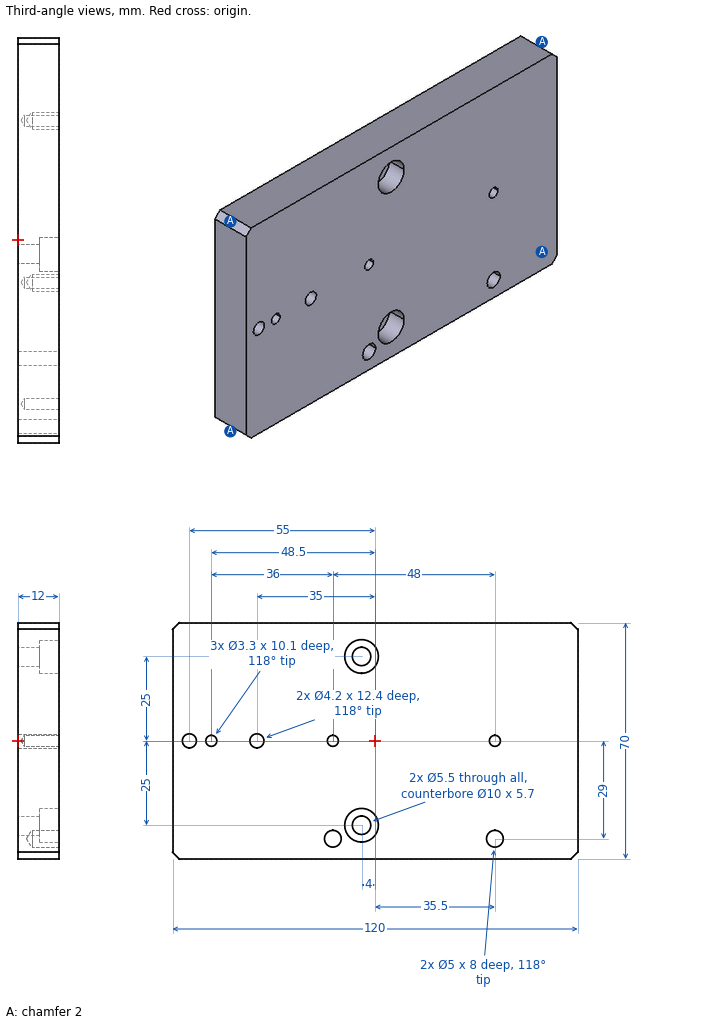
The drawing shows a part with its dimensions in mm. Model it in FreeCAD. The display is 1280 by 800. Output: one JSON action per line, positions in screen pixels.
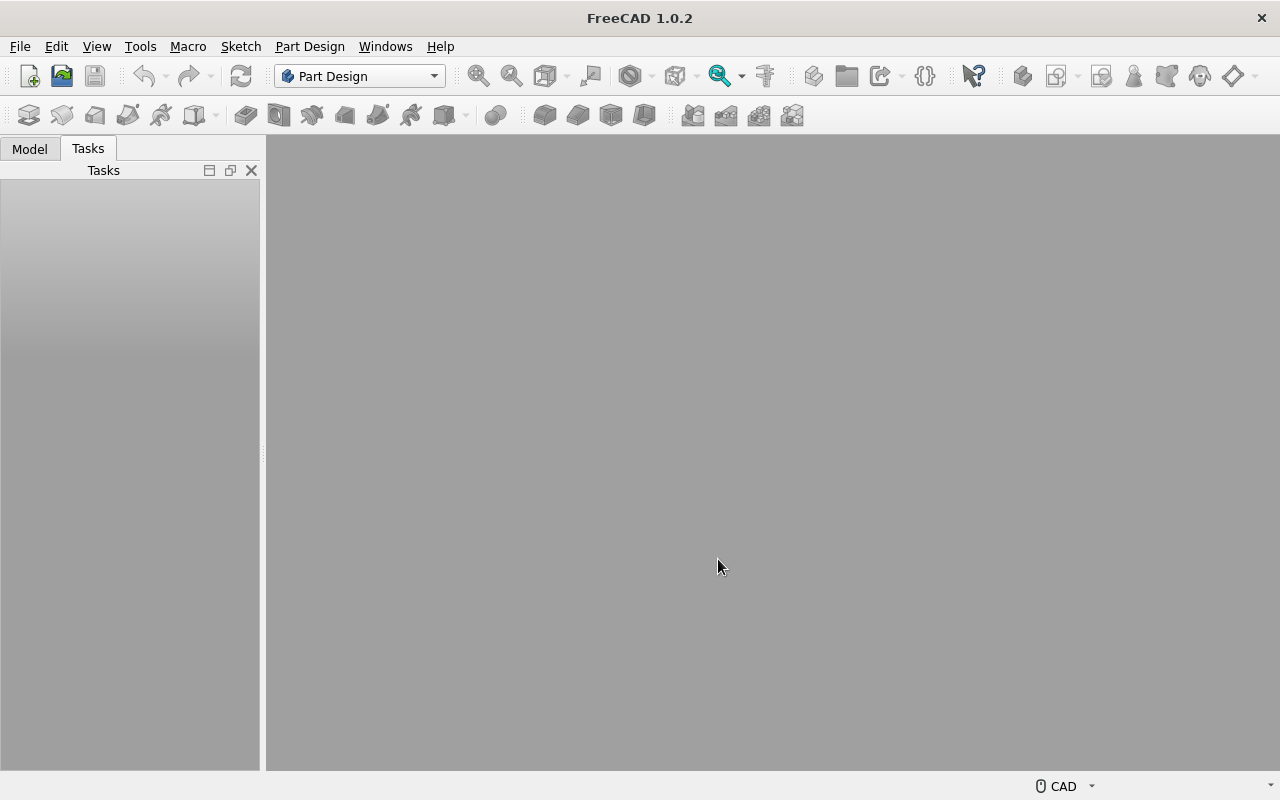
{"action": "left_click", "coordinate": [29, 76]}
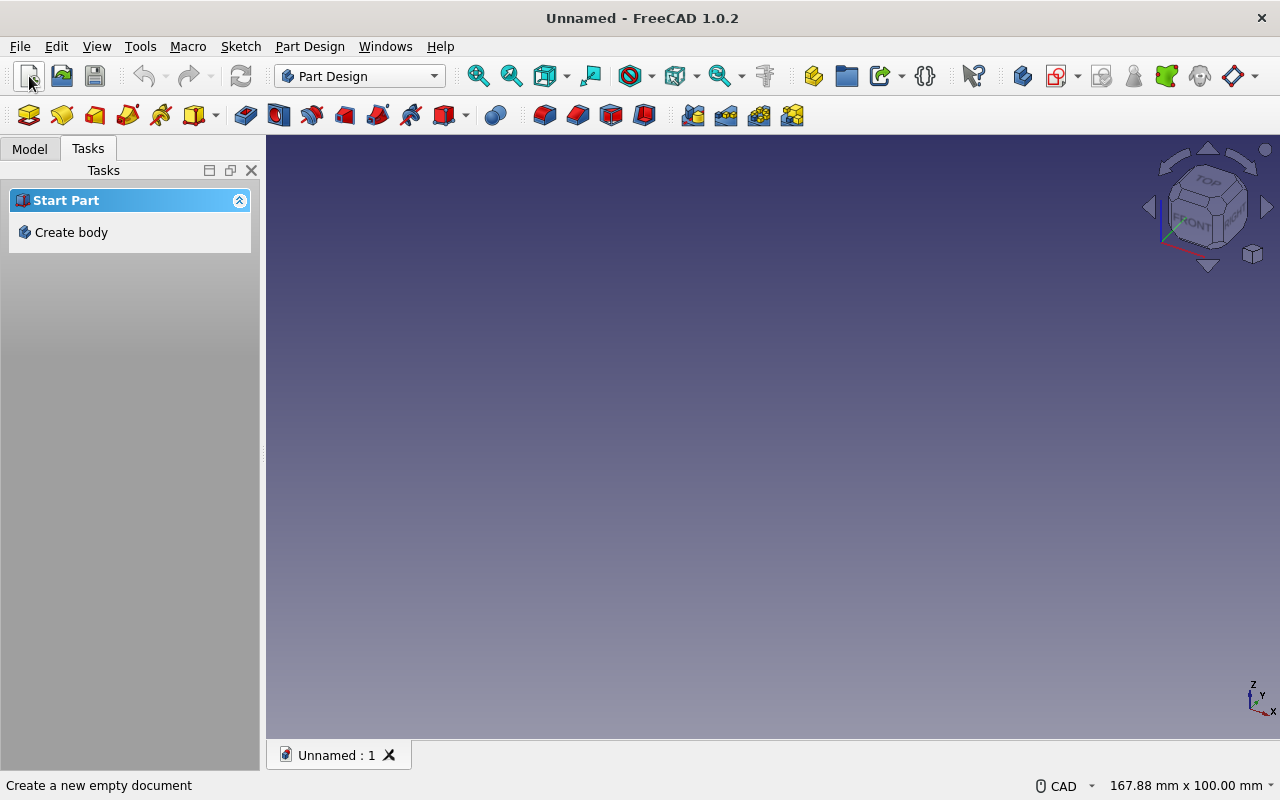
{"action": "left_click", "coordinate": [1056, 76]}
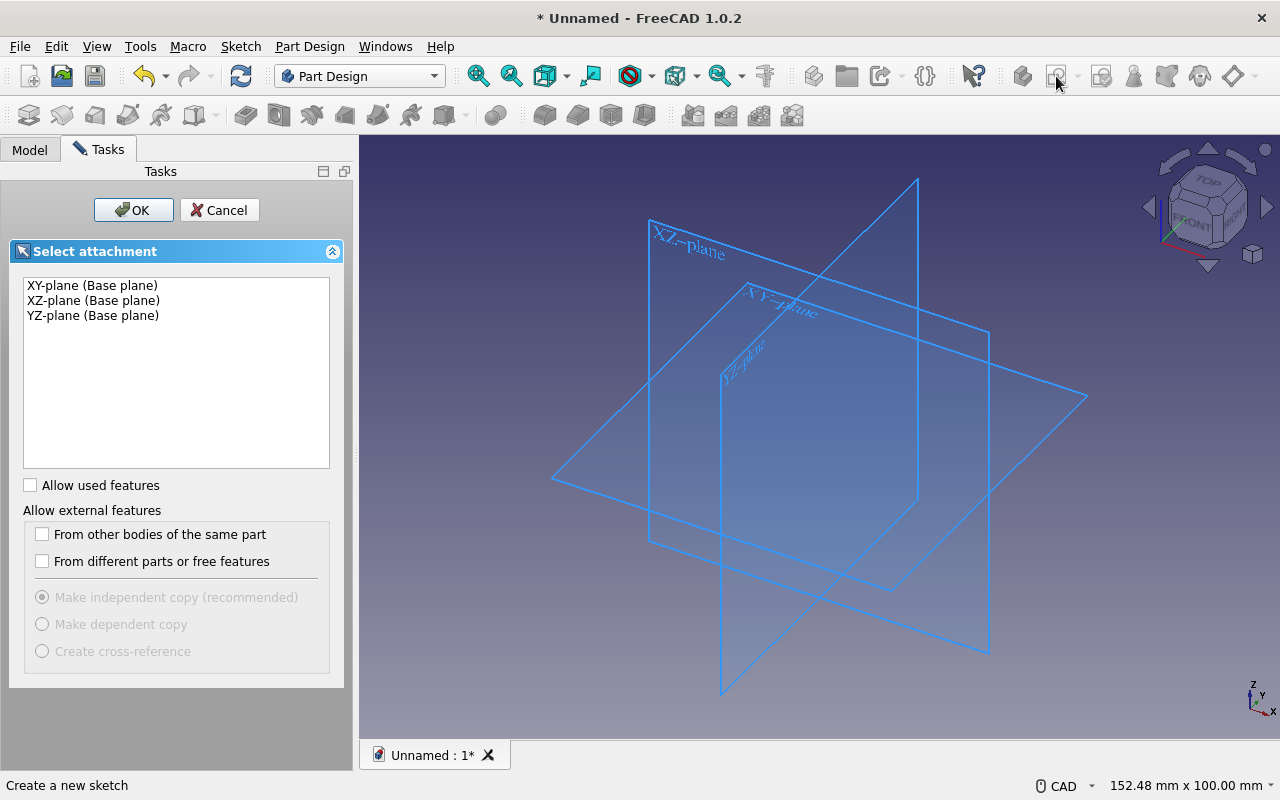
{"action": "left_click", "coordinate": [84, 316]}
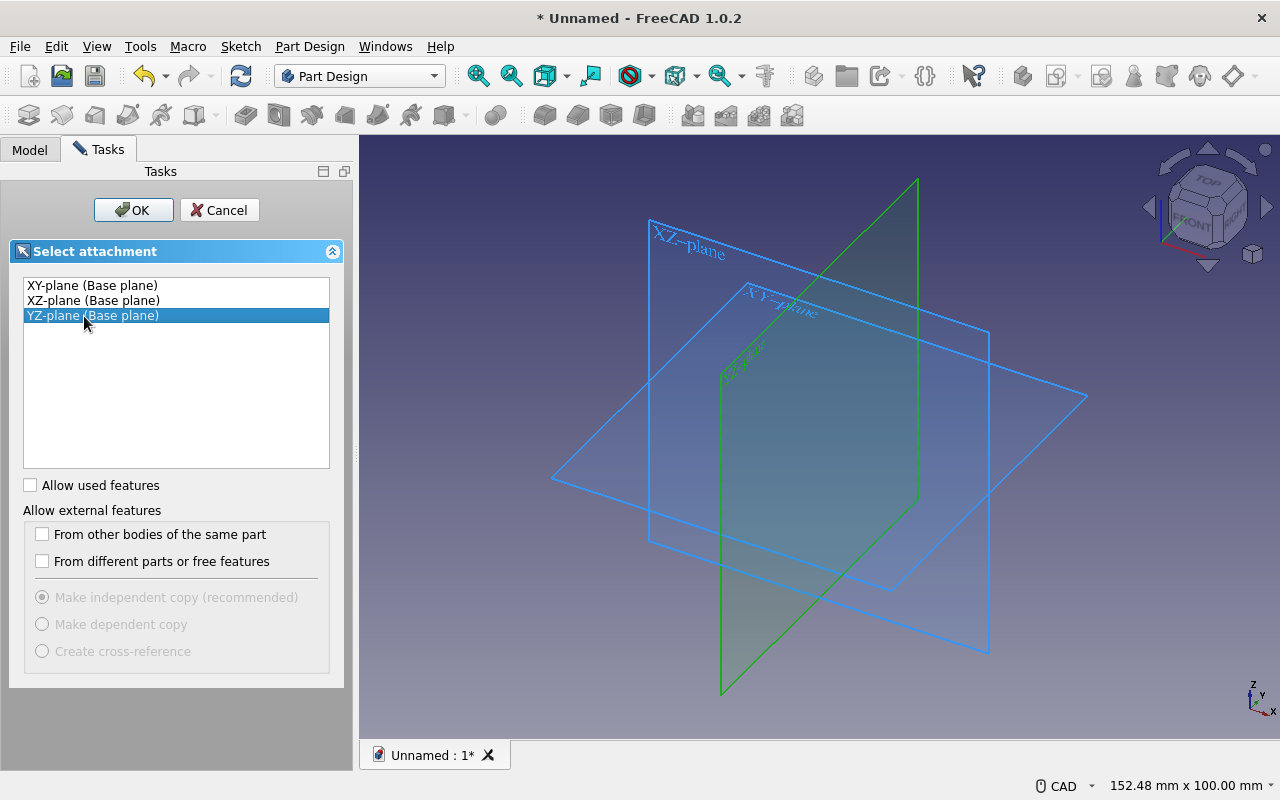
{"action": "left_click", "coordinate": [134, 210]}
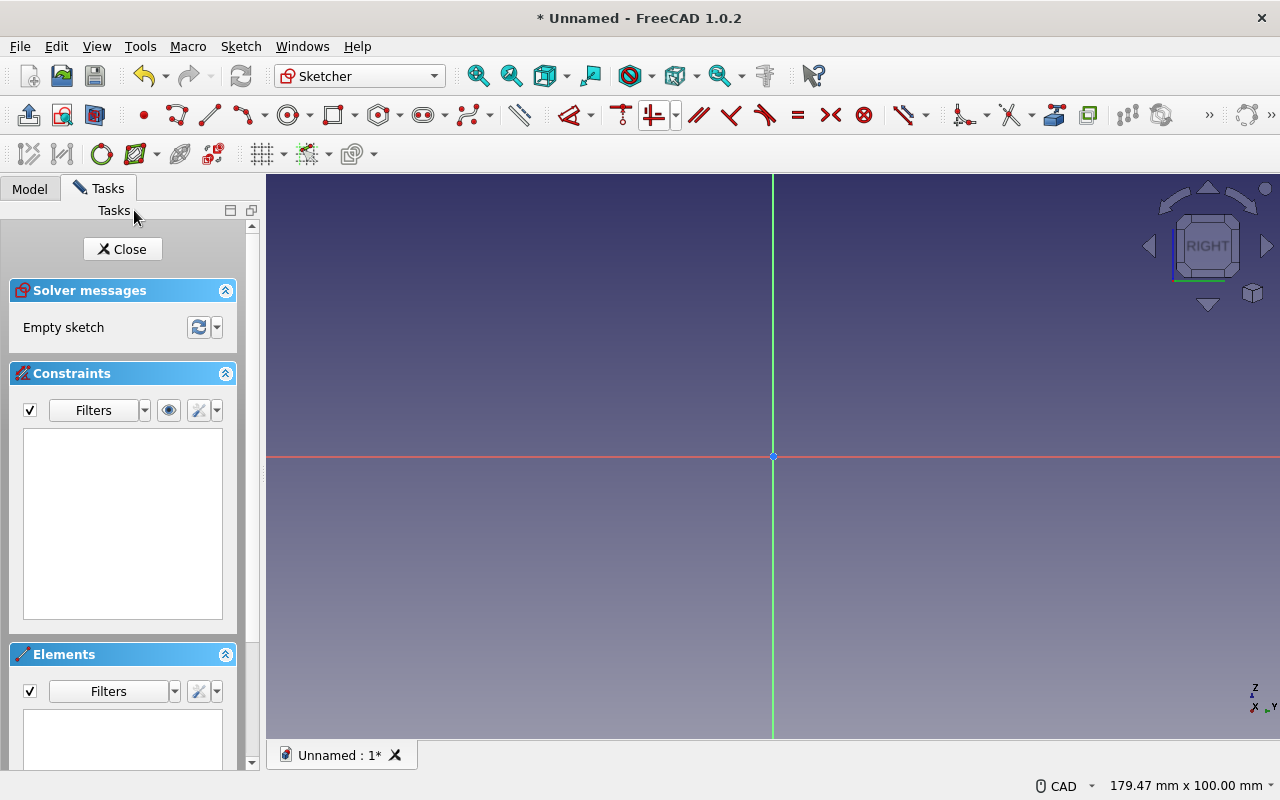
{"action": "scroll", "coordinate": [395, 456], "scroll_direction": "down", "scroll_amount": 1}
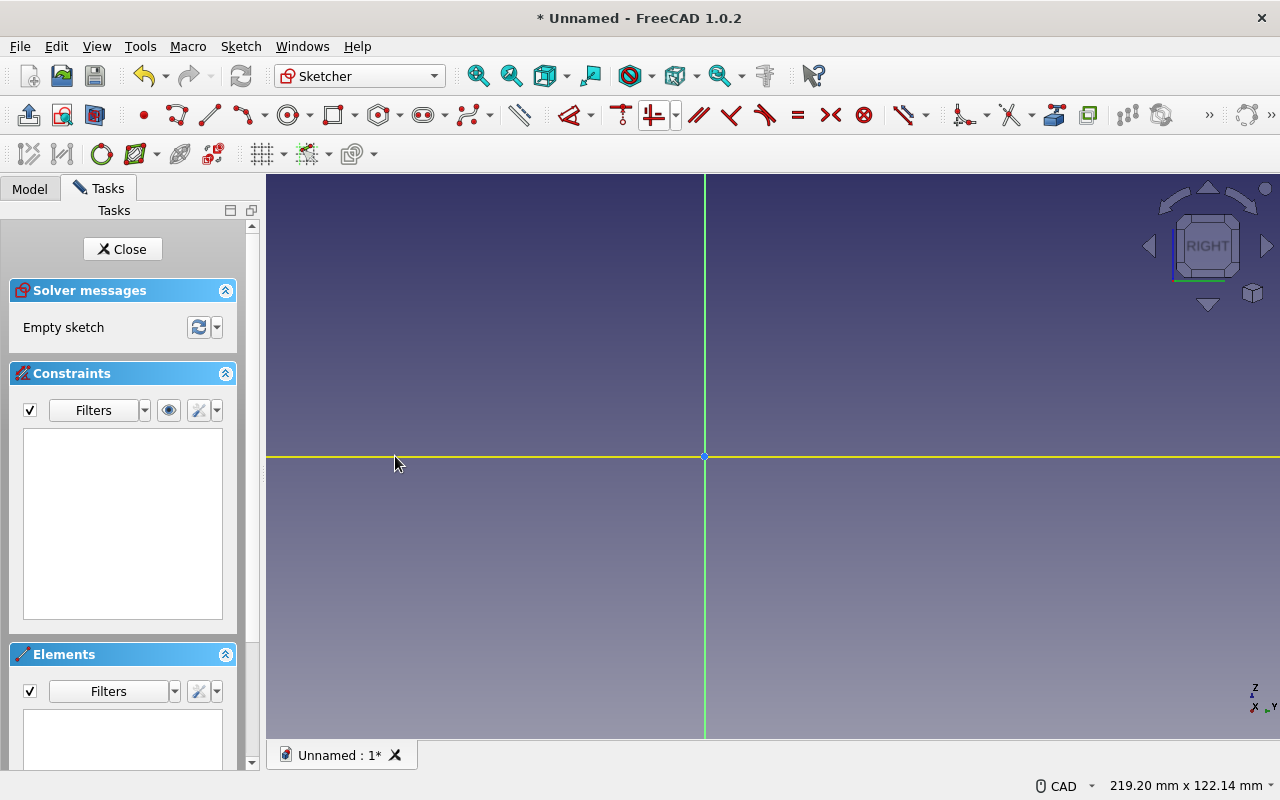
{"action": "key", "text": "g v"}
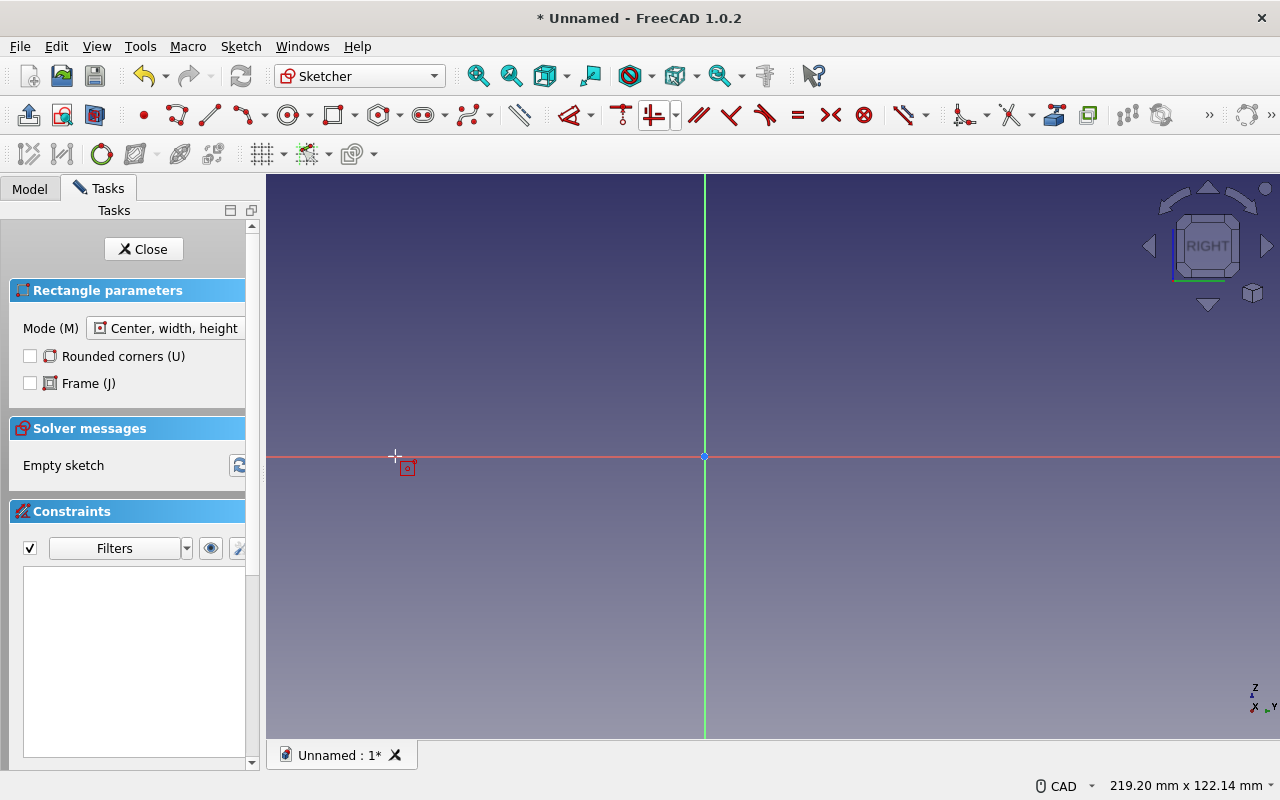
{"action": "left_click", "coordinate": [705, 456]}
{"action": "left_click", "coordinate": [982, 295]}
{"action": "key", "text": "Escape"}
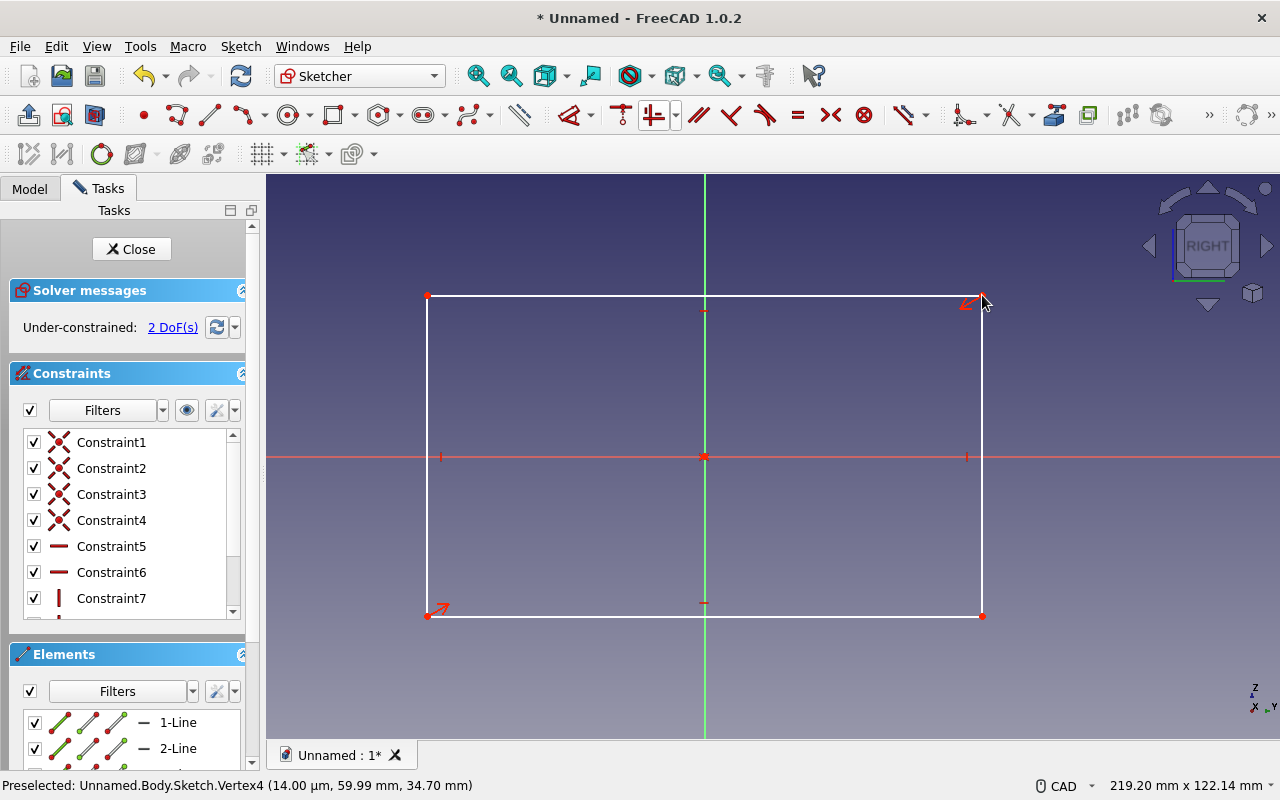
{"action": "left_click", "coordinate": [568, 116]}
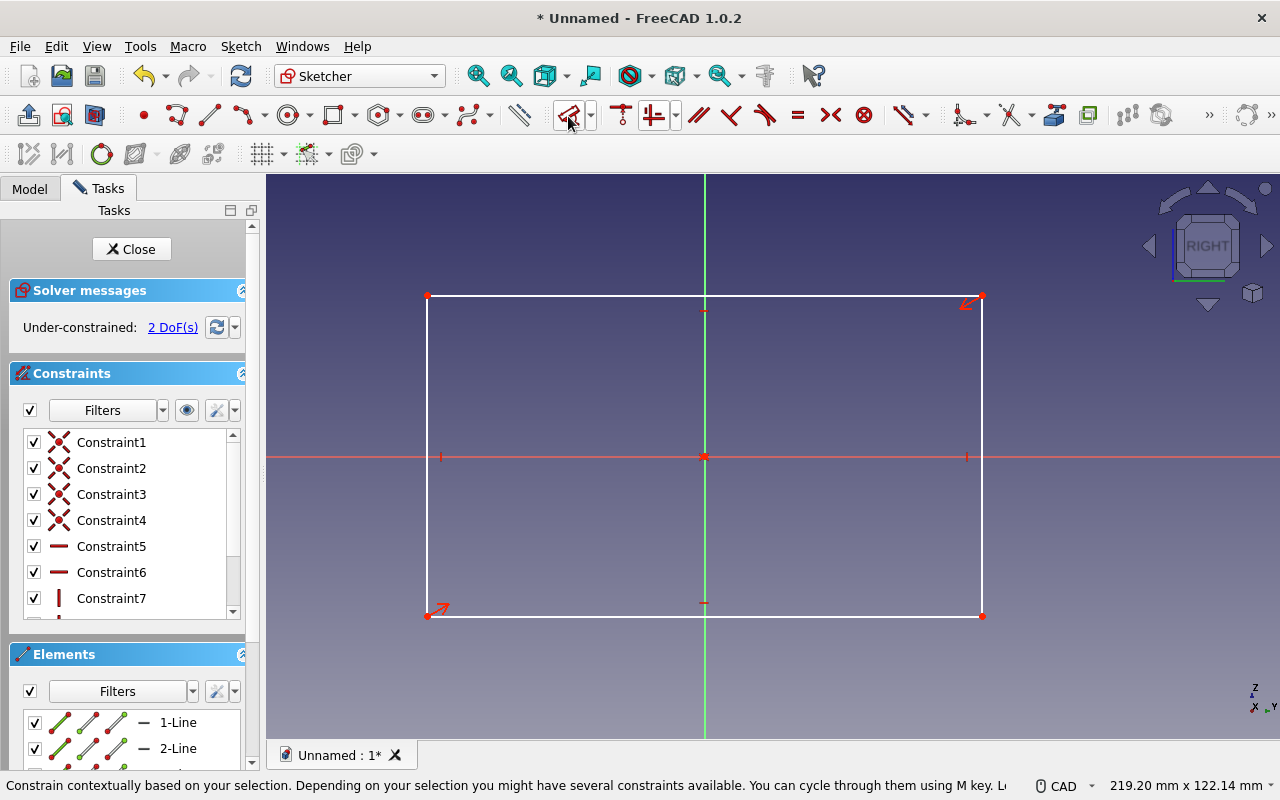
{"action": "left_click", "coordinate": [982, 521]}
{"action": "left_click", "coordinate": [1016, 383]}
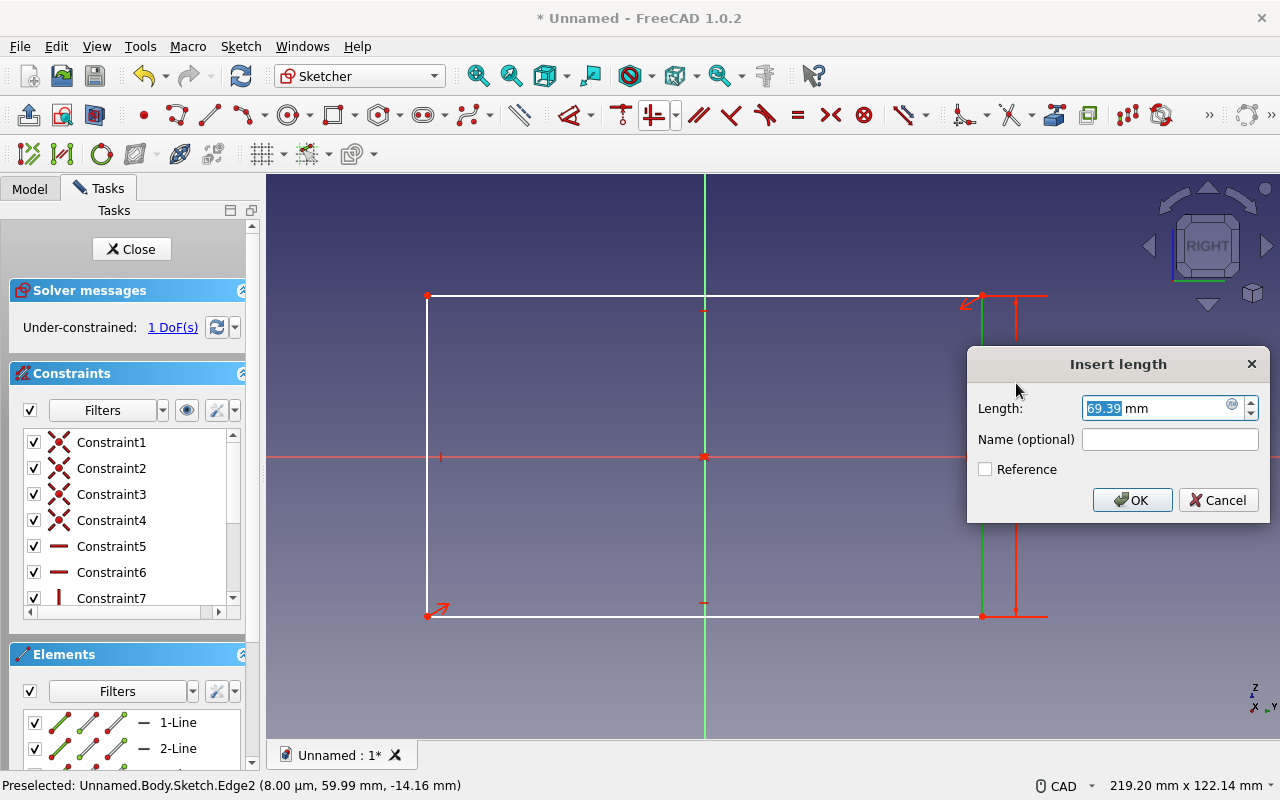
{"action": "type", "text": "70"}
{"action": "key", "text": "Return"}